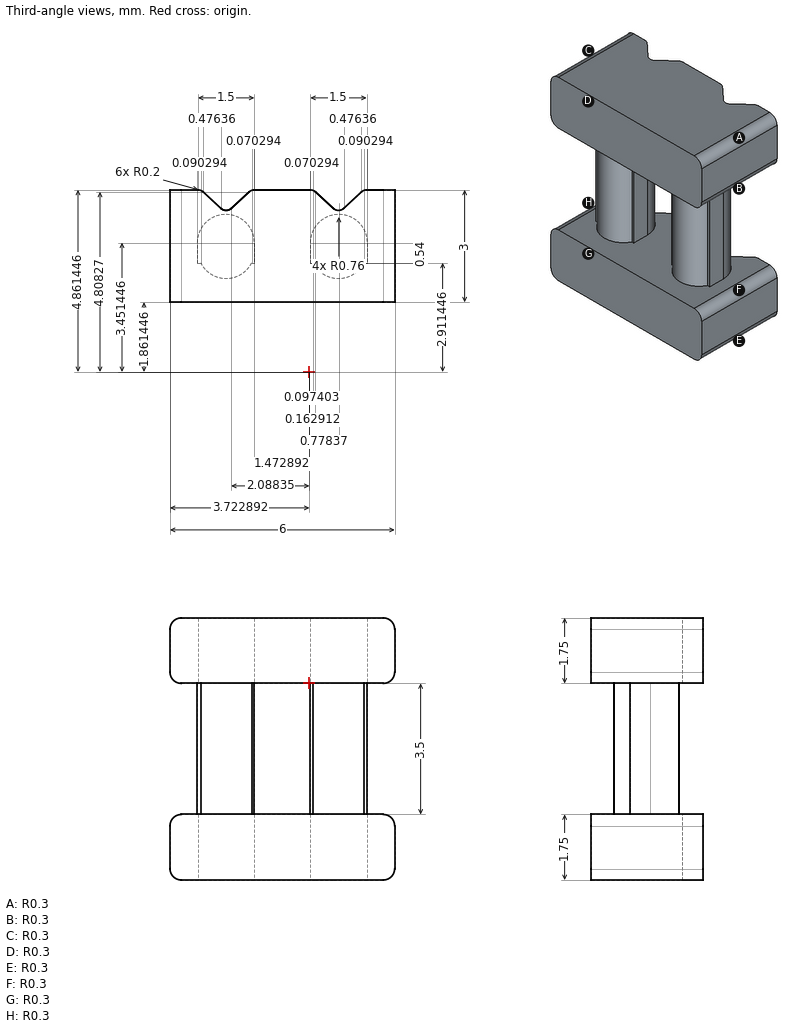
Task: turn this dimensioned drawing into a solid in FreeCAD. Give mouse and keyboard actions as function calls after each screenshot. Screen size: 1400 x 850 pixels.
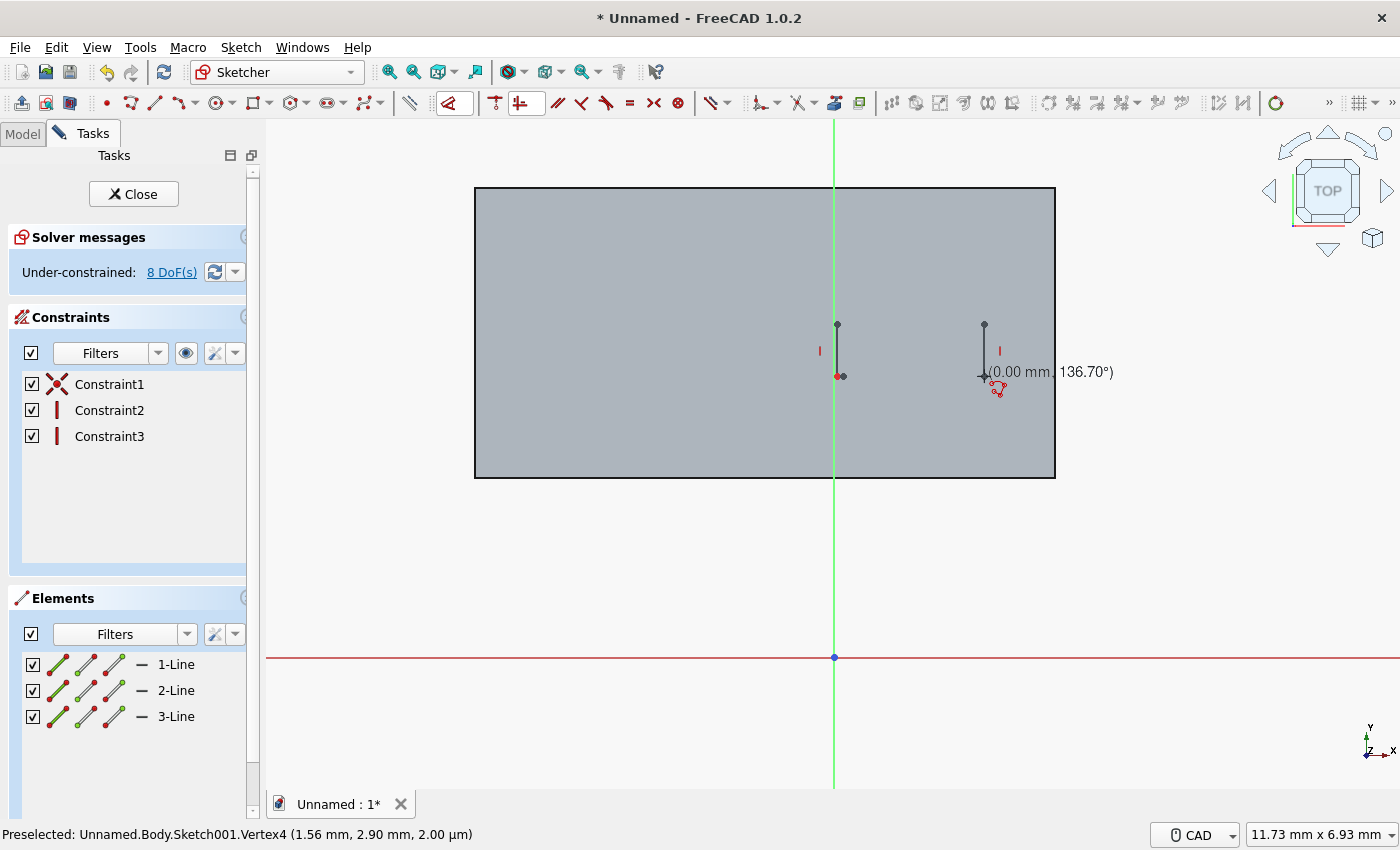
scroll(975, 376, up, 3)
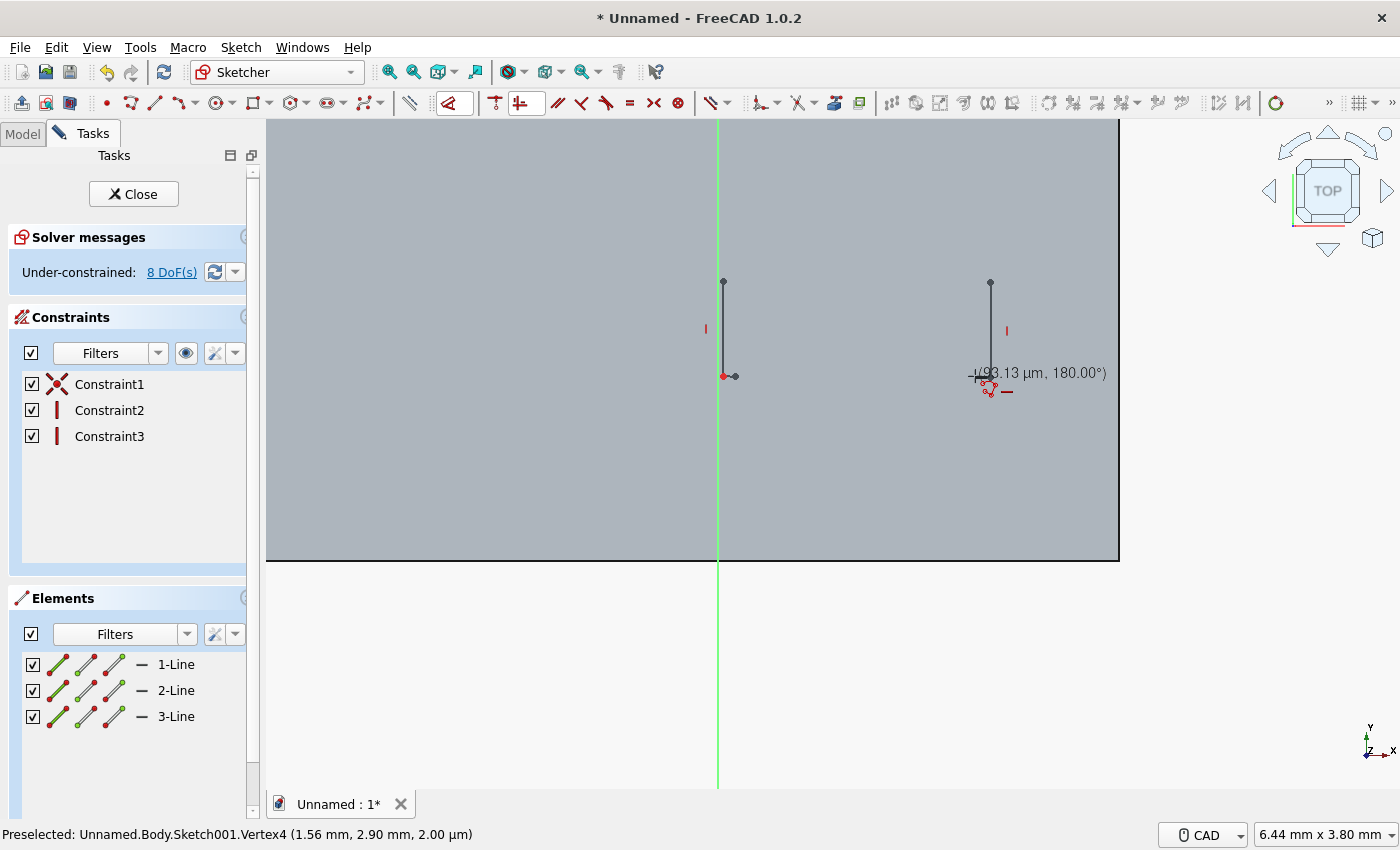
click(975, 376)
right_click(975, 376)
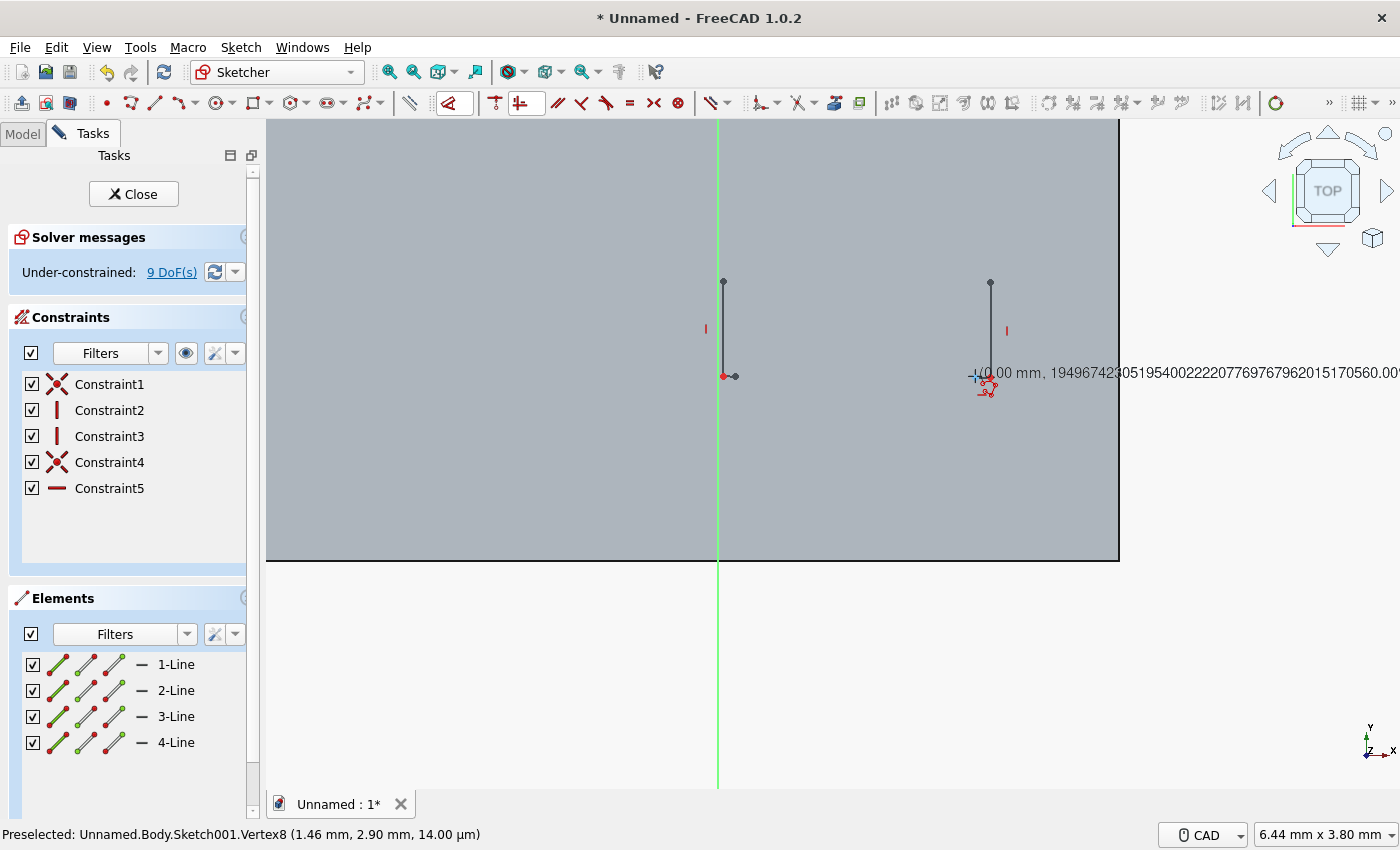
click(180, 104)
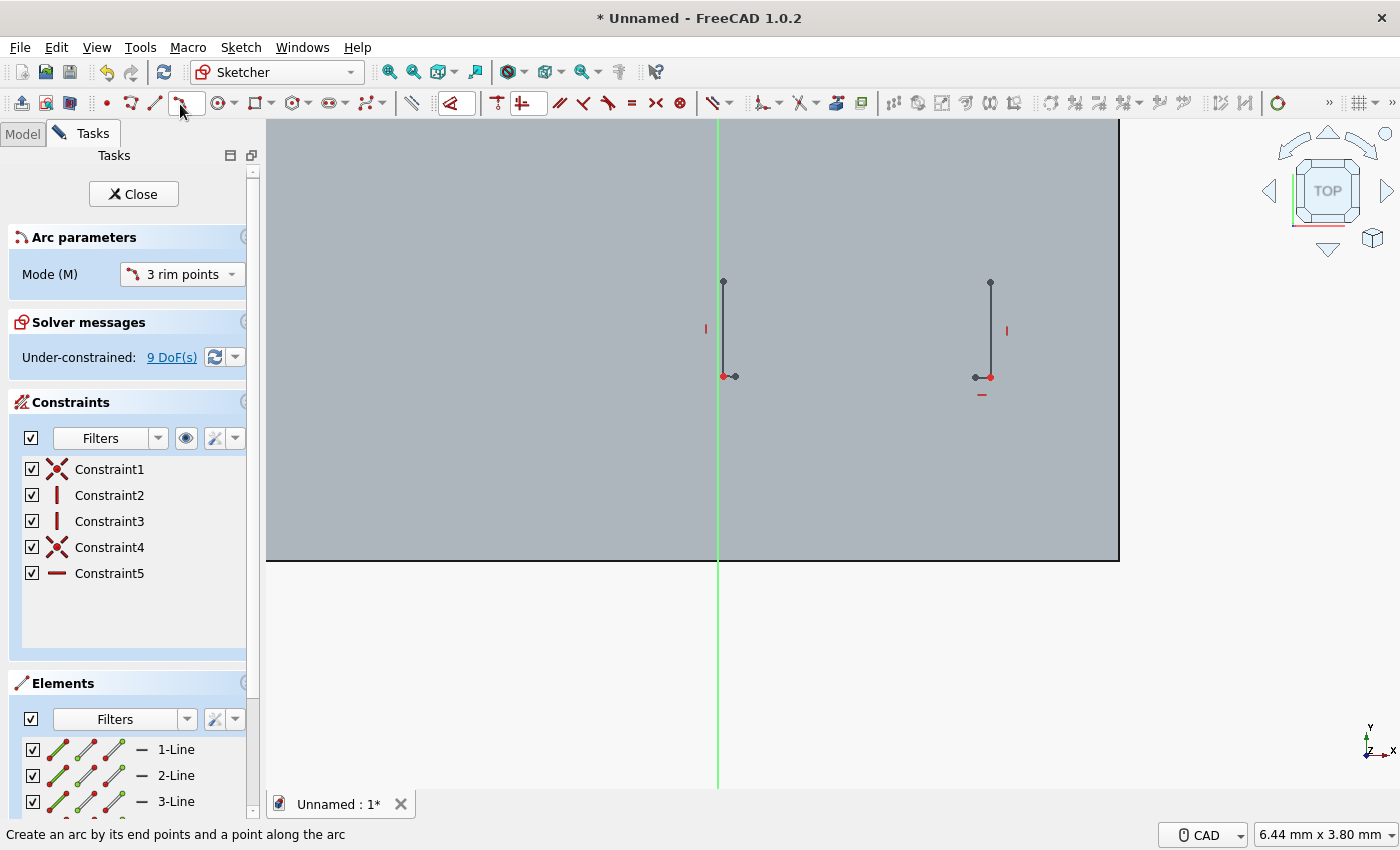
scroll(723, 281, up, 7)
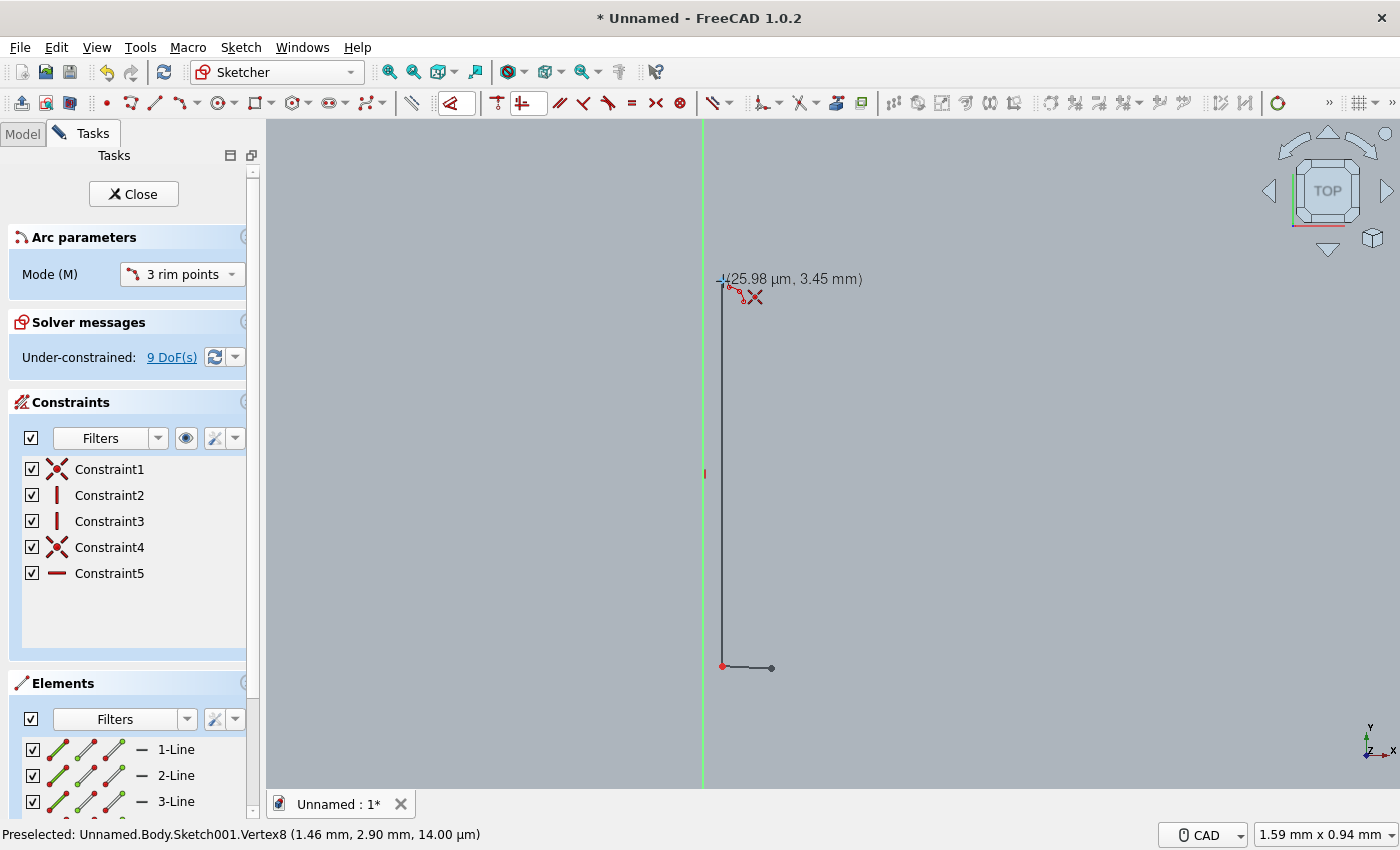
click(722, 281)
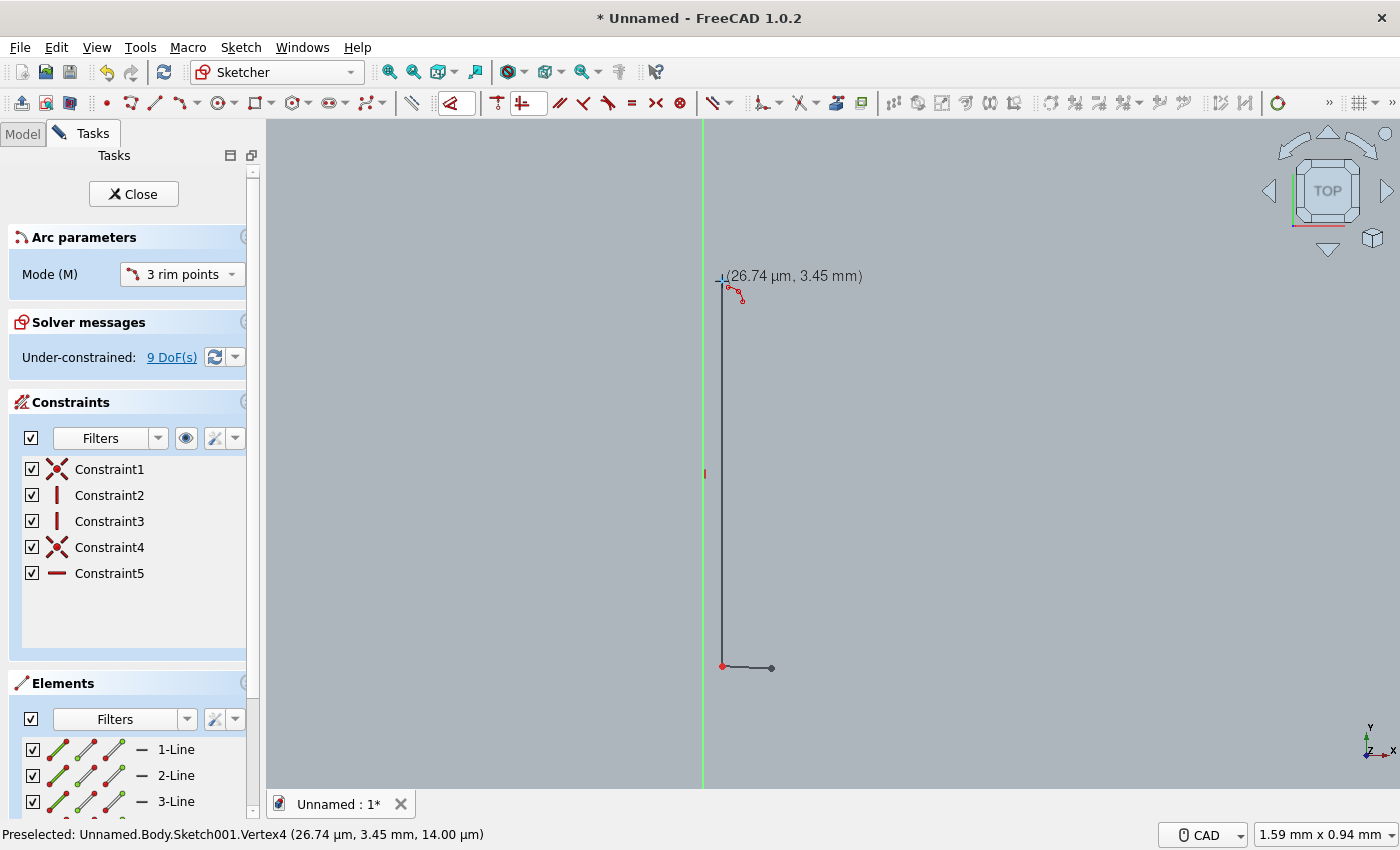
scroll(855, 331, down, 10)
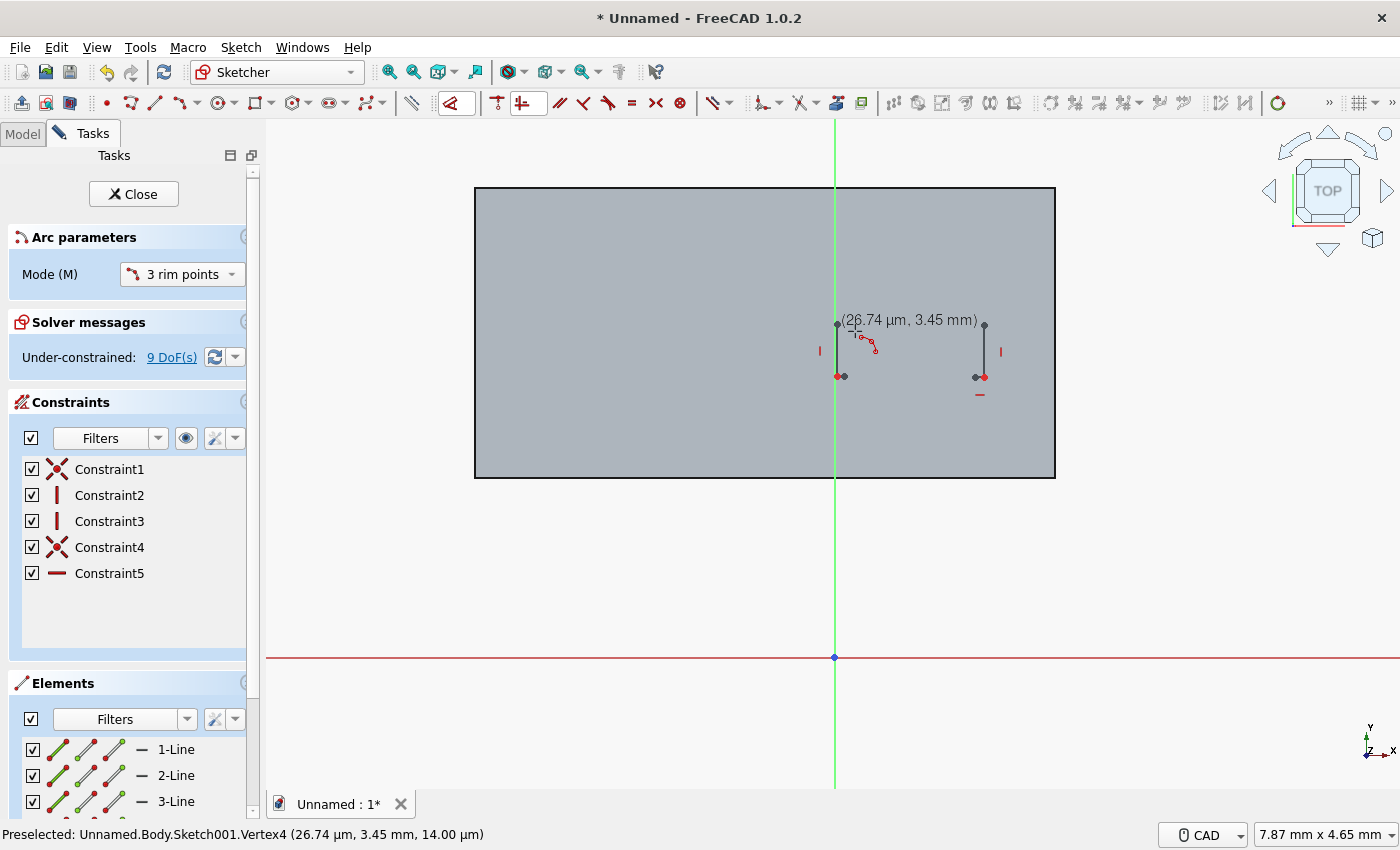
click(984, 325)
click(911, 251)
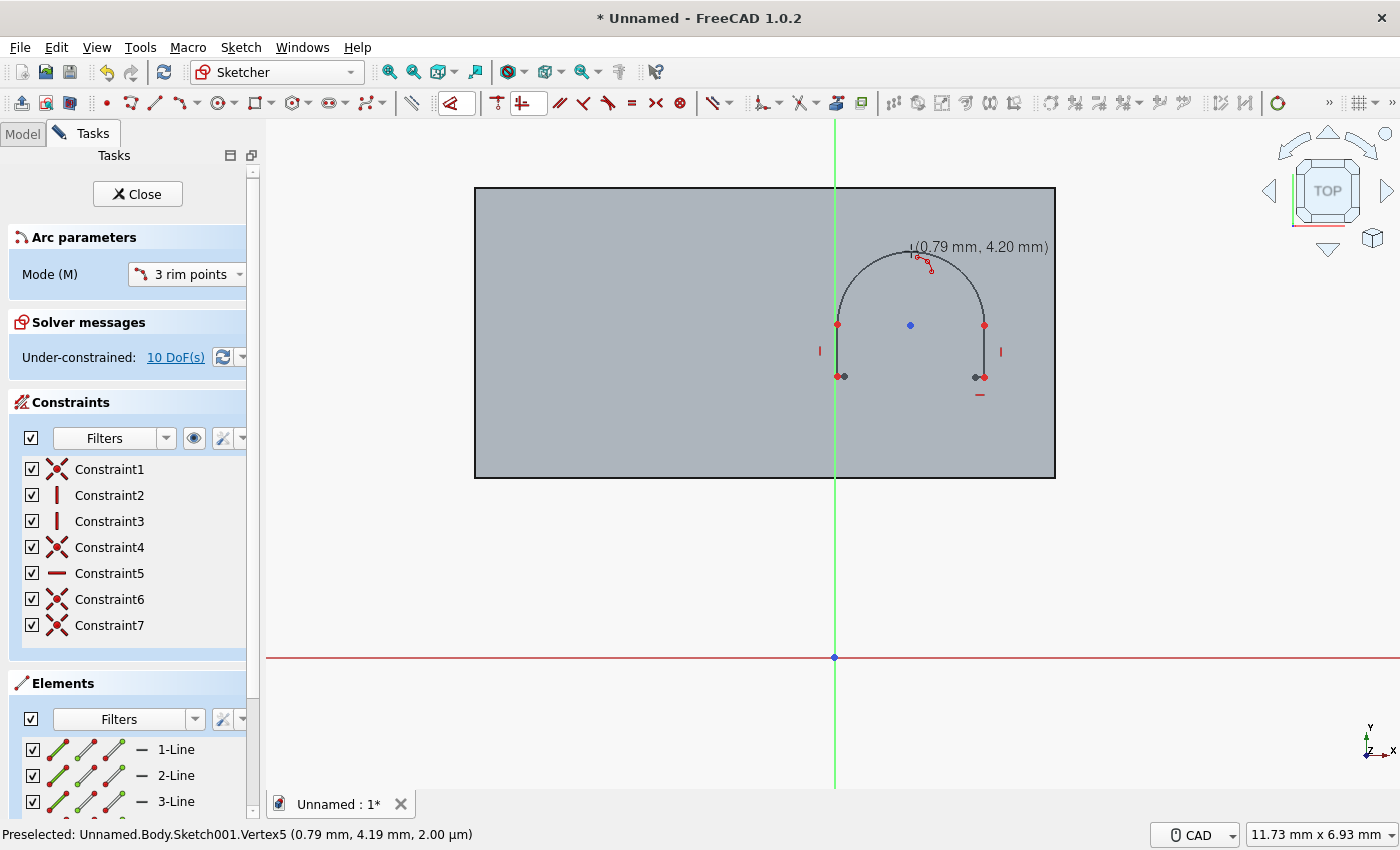
scroll(976, 377, up, 7)